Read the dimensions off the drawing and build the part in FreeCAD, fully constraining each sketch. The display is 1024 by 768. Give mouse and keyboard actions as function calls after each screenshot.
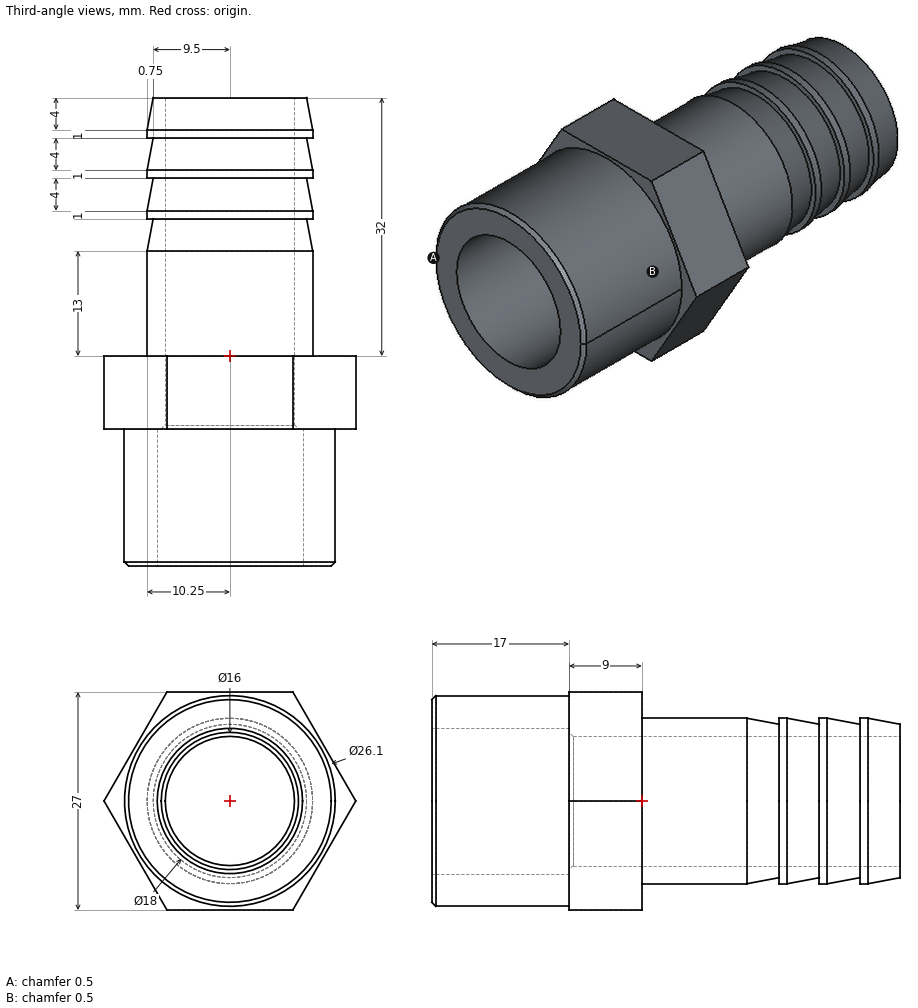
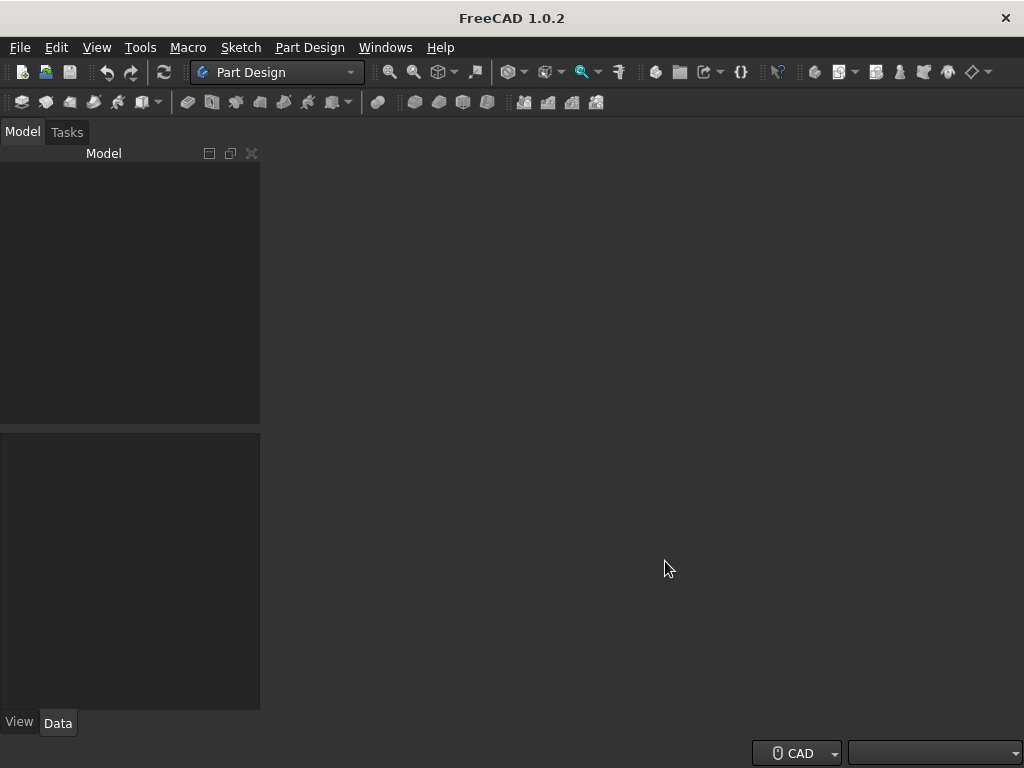
key(ctrl+n)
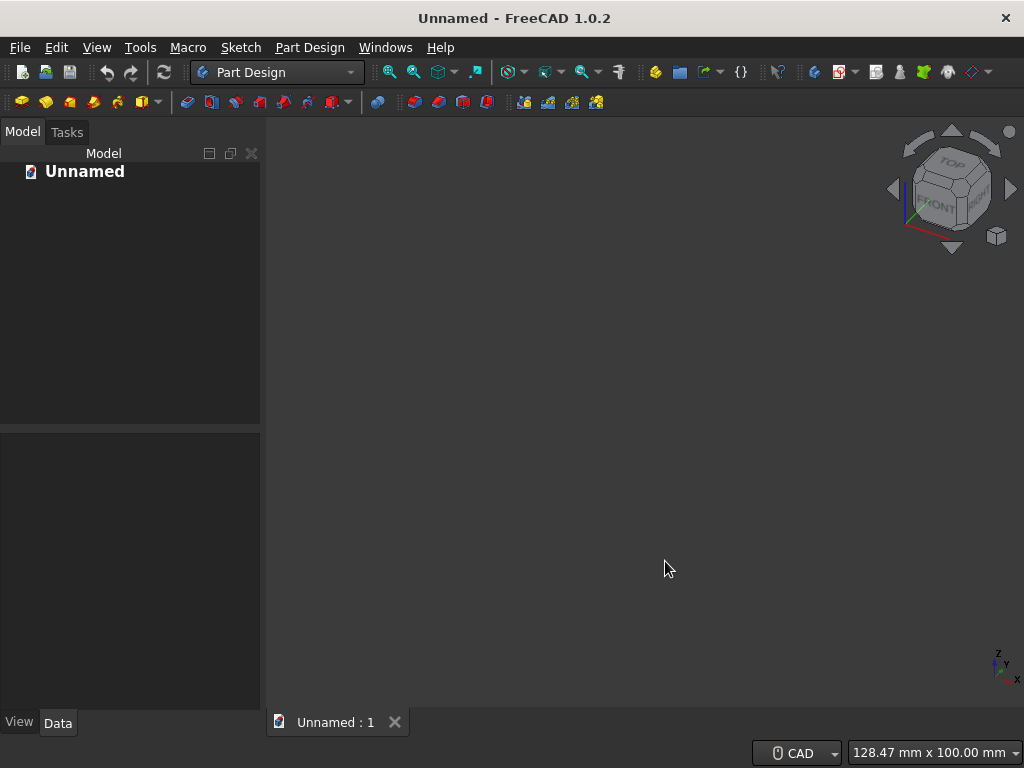
click(840, 72)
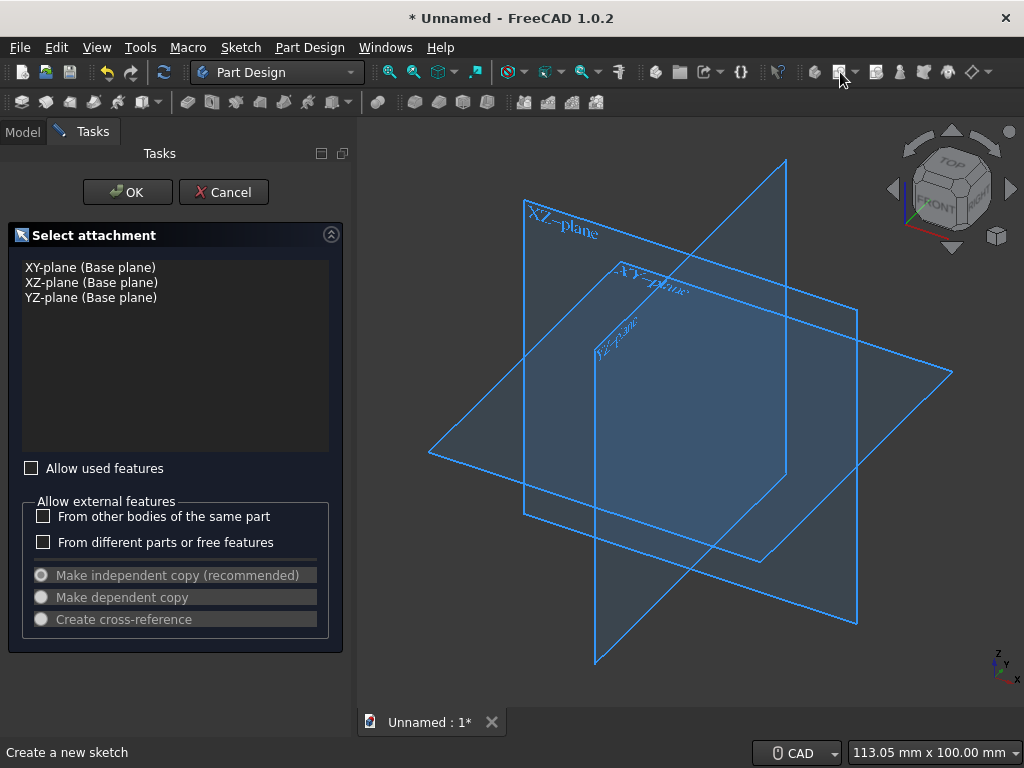
click(82, 268)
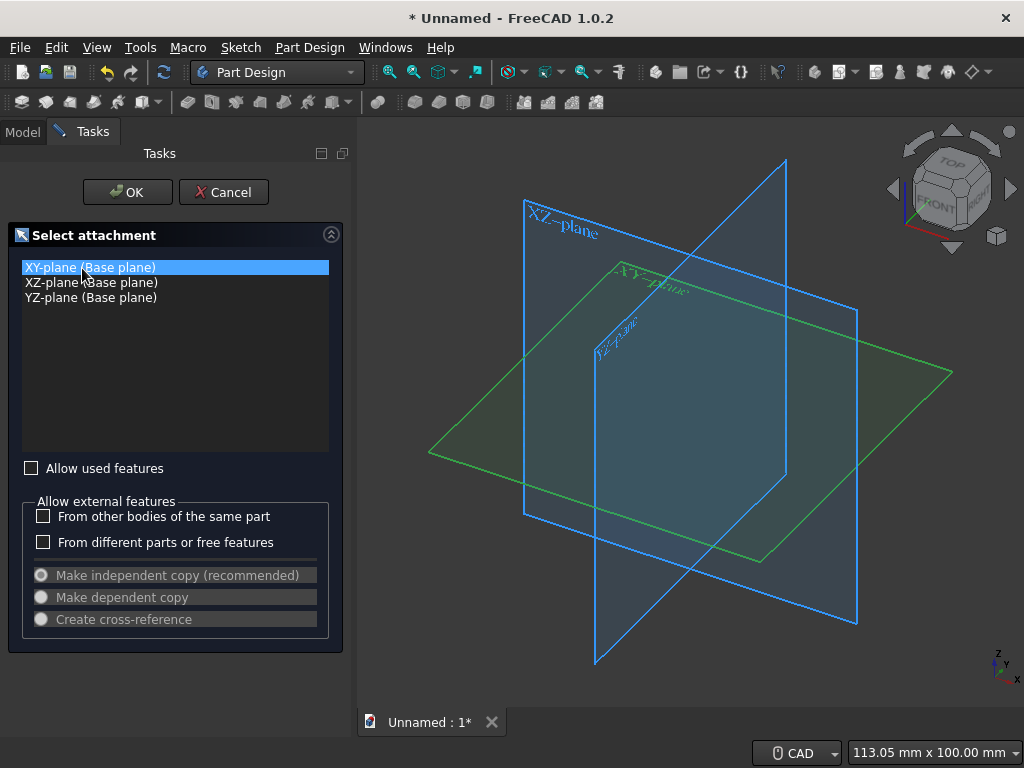
click(128, 192)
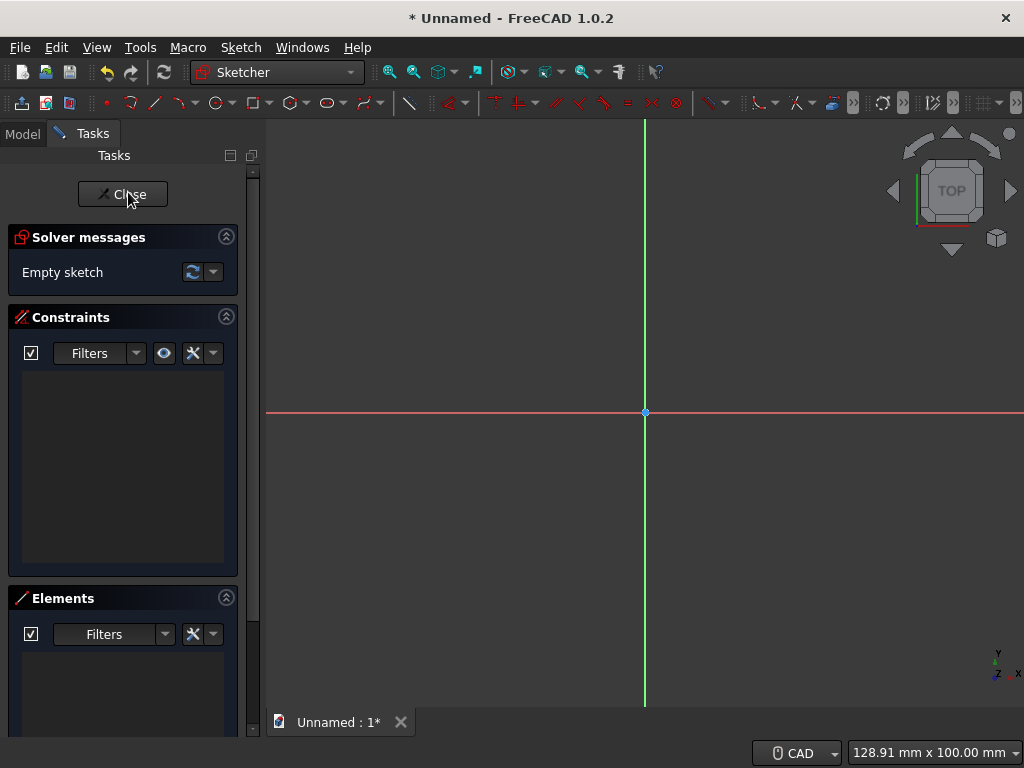
scroll(662, 204, up, 3)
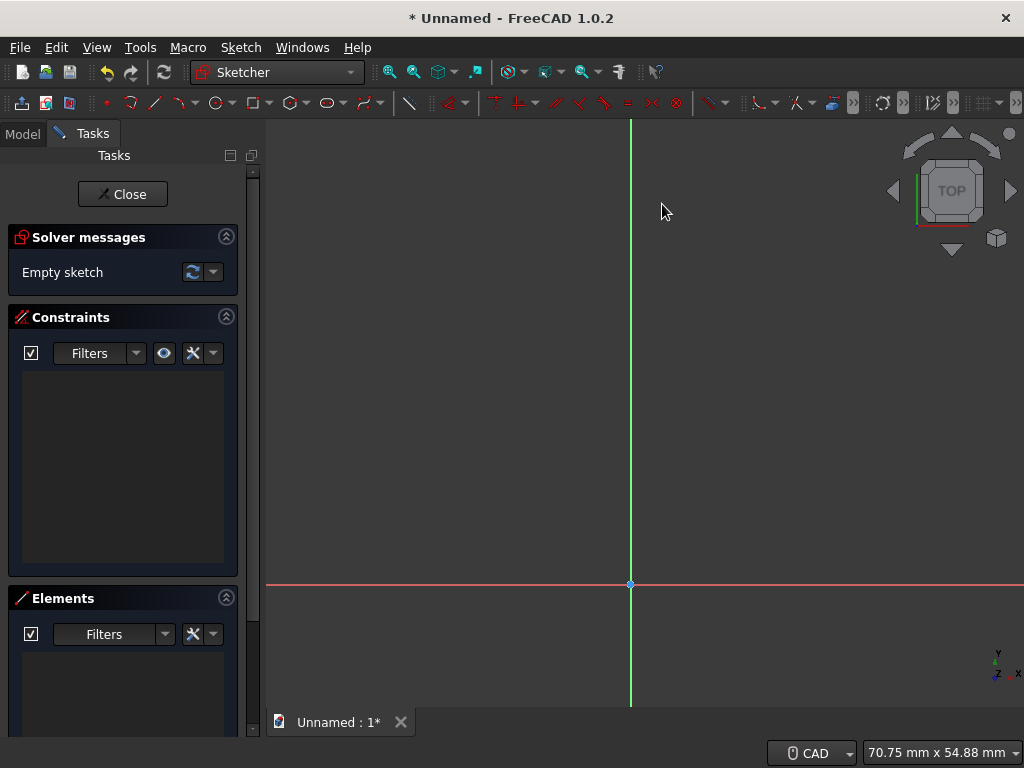
key(g)
key(m)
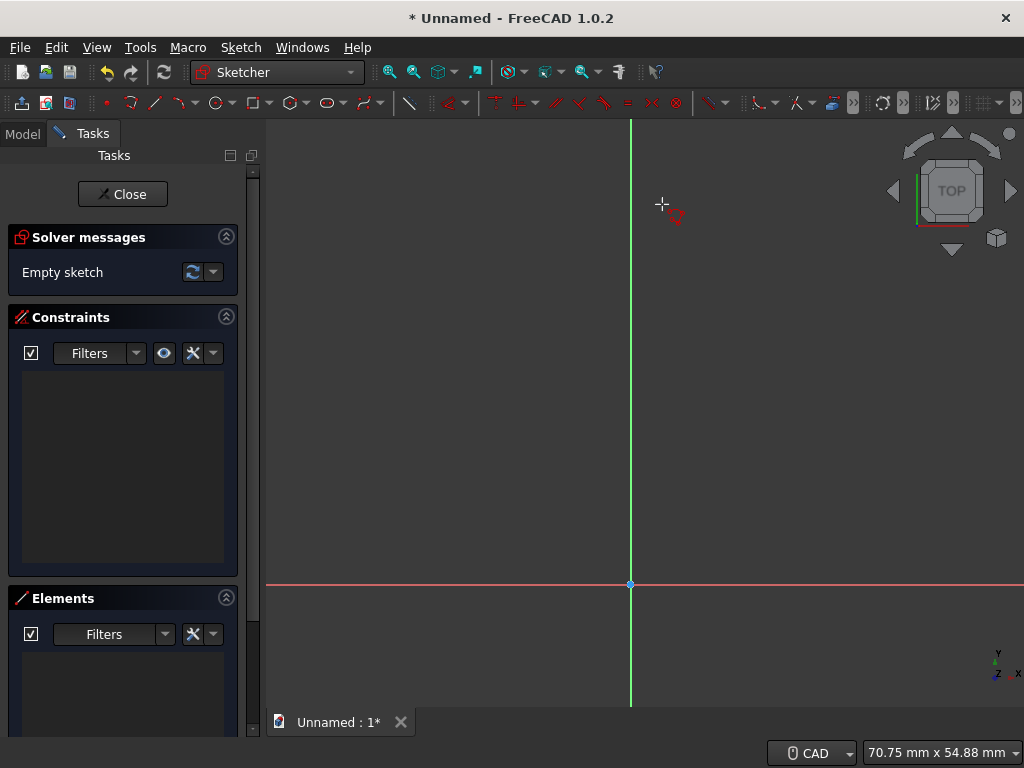
click(631, 585)
click(622, 242)
click(529, 242)
click(521, 285)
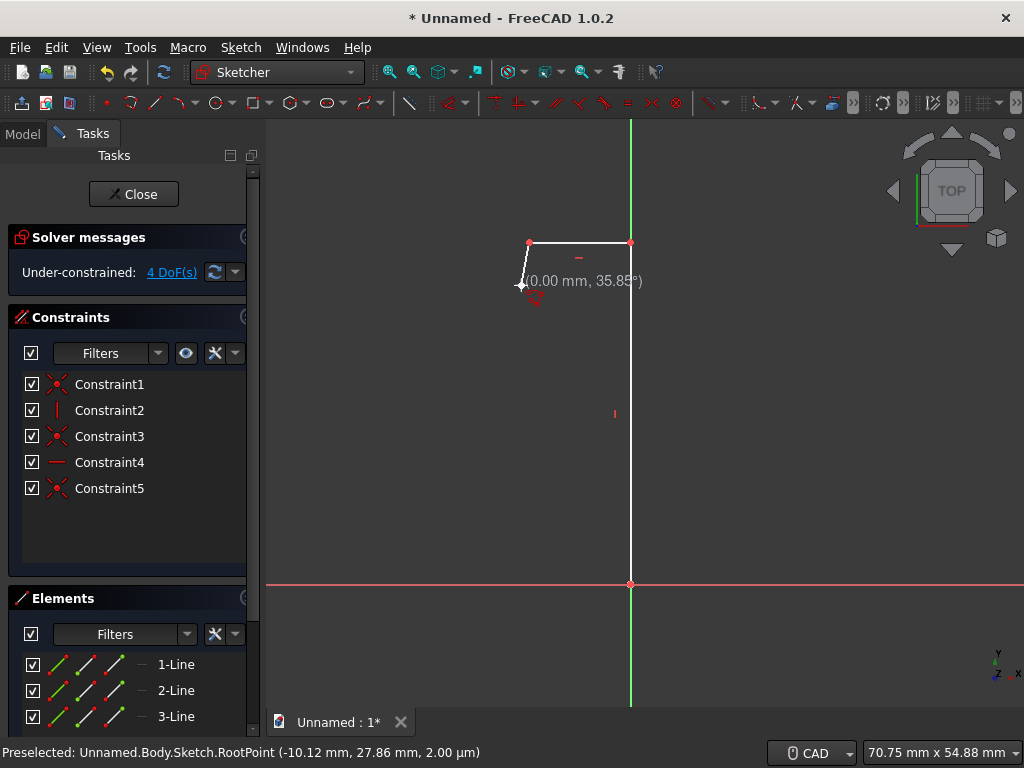
scroll(521, 295, up, 2)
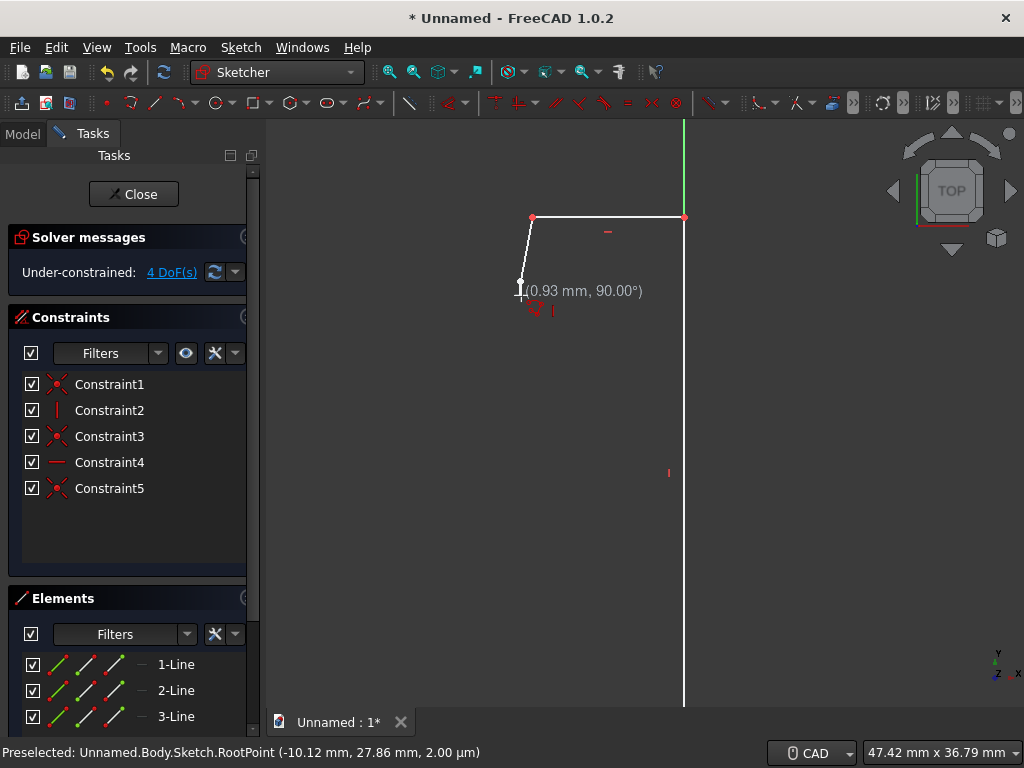
click(521, 295)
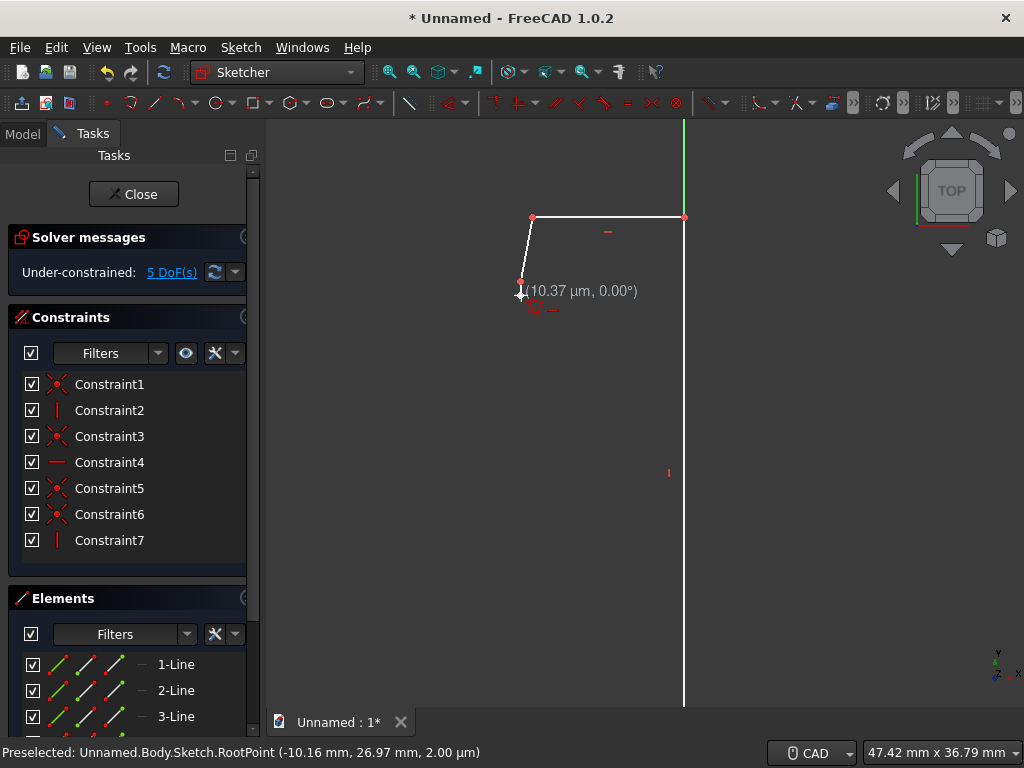
scroll(532, 295, up, 2)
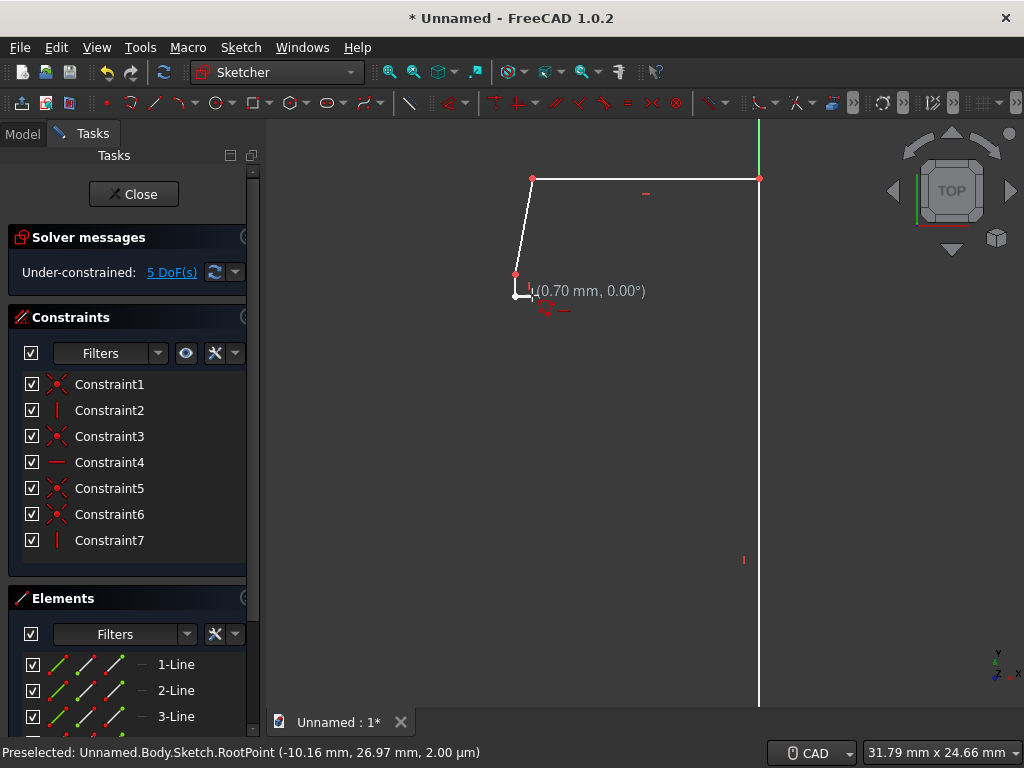
click(533, 295)
click(515, 391)
click(515, 415)
click(533, 415)
click(515, 510)
click(515, 534)
click(533, 534)
click(515, 629)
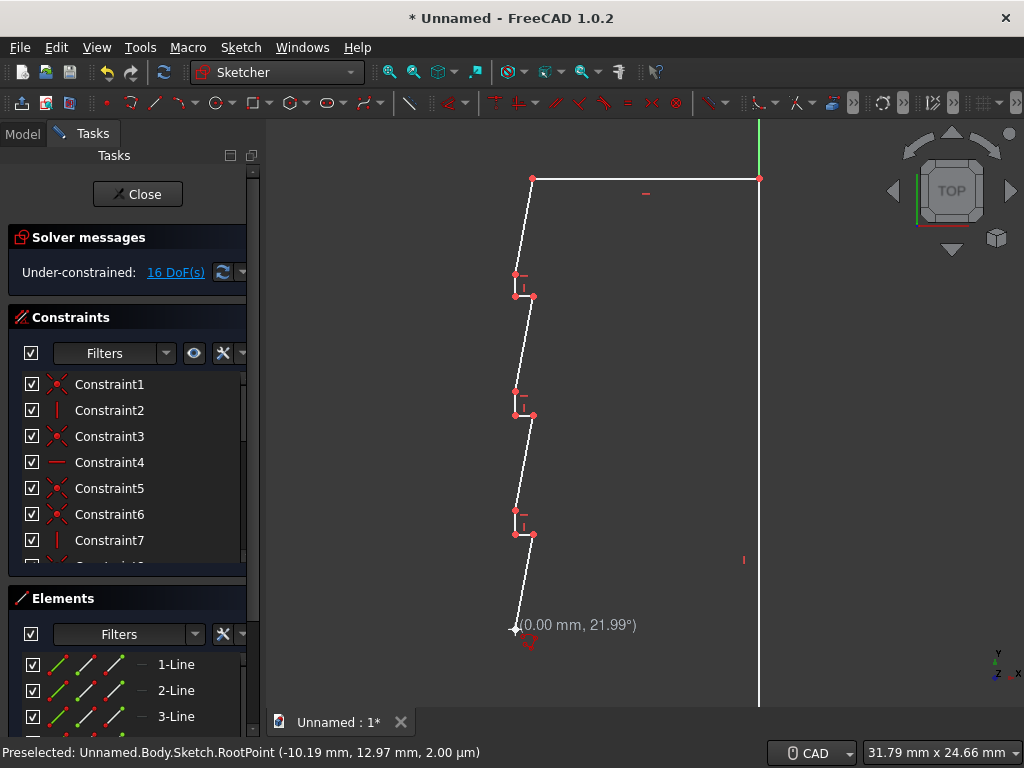
scroll(527, 295, down, 4)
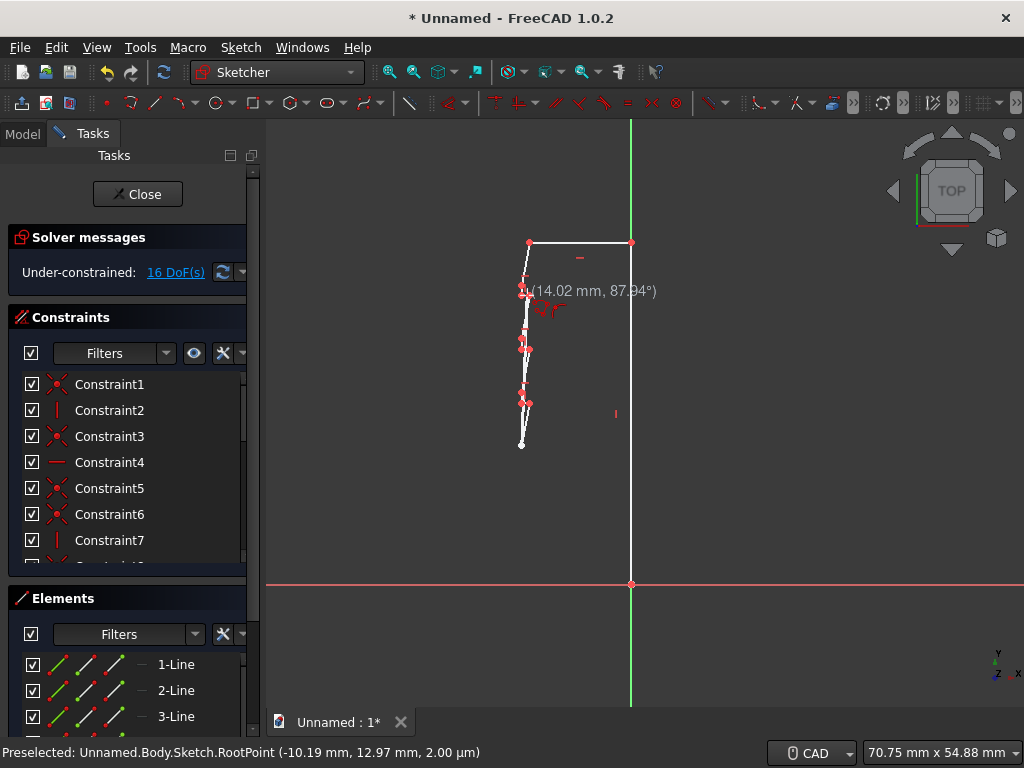
click(522, 576)
click(631, 585)
key(Escape)
key(Escape)